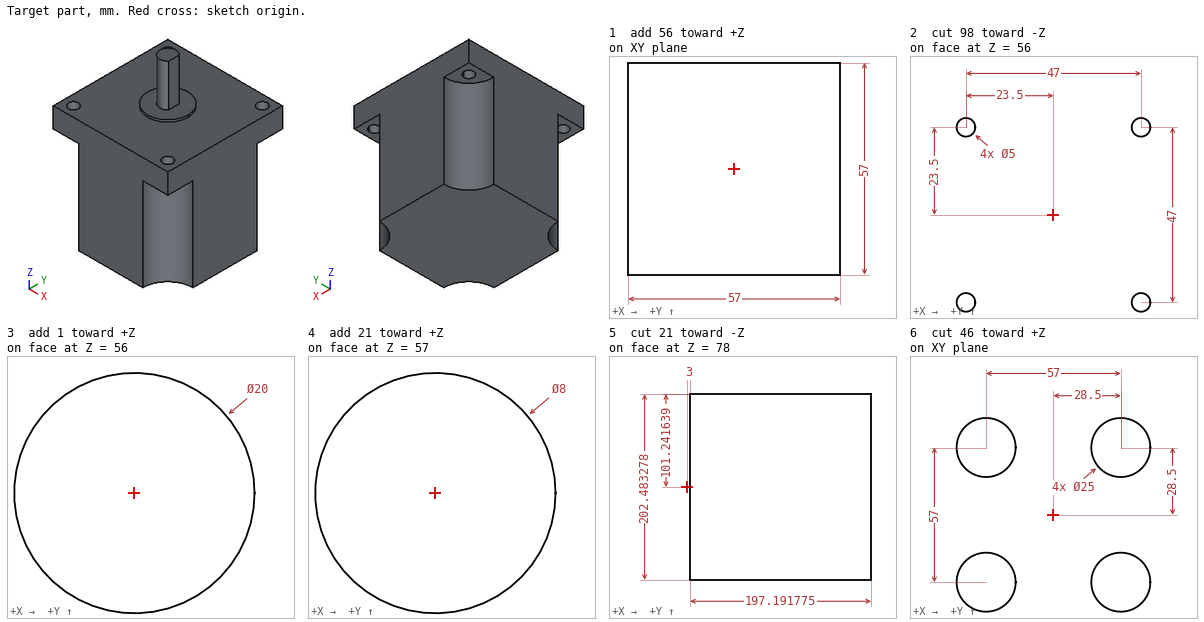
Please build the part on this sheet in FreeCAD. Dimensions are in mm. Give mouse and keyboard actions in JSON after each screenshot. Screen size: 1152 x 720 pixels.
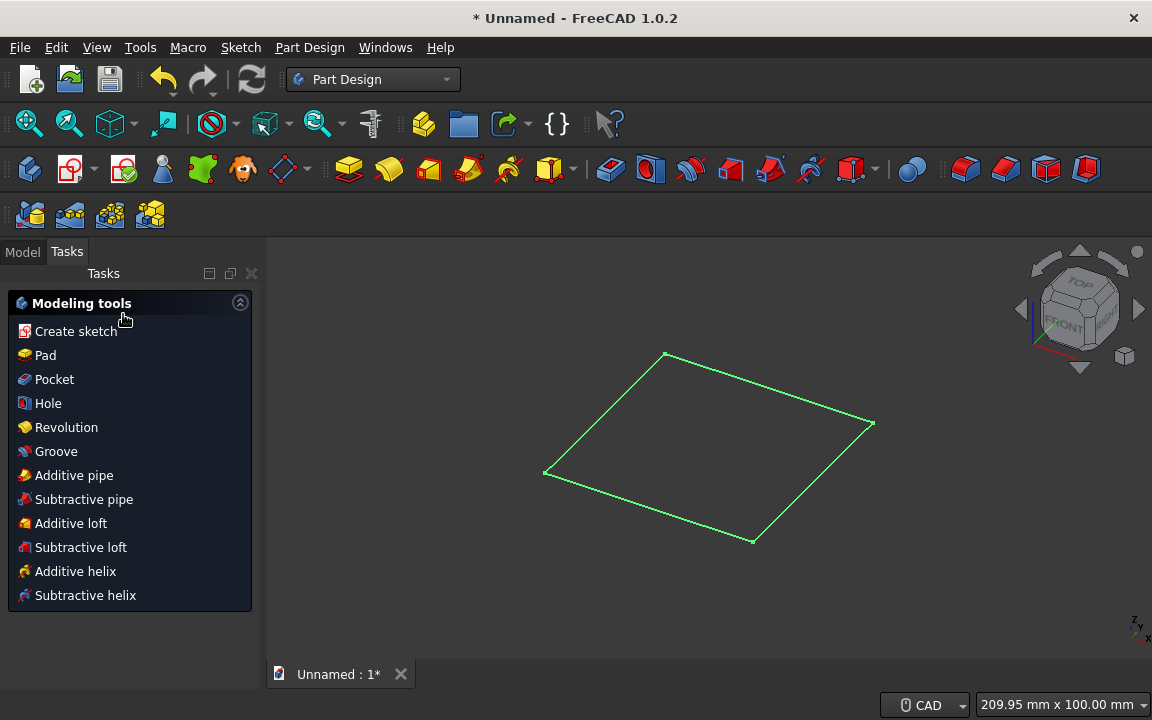
{"action": "left_click", "coordinate": [350, 170]}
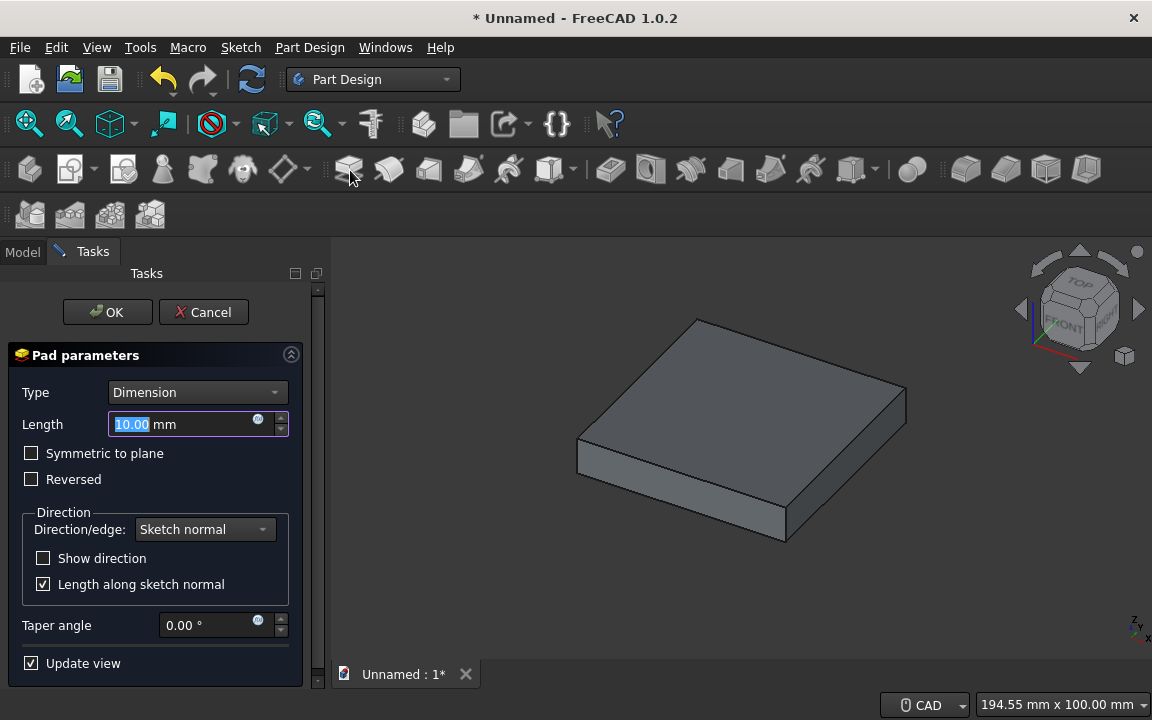
{"action": "type", "text": "56"}
{"action": "key", "text": "Tab"}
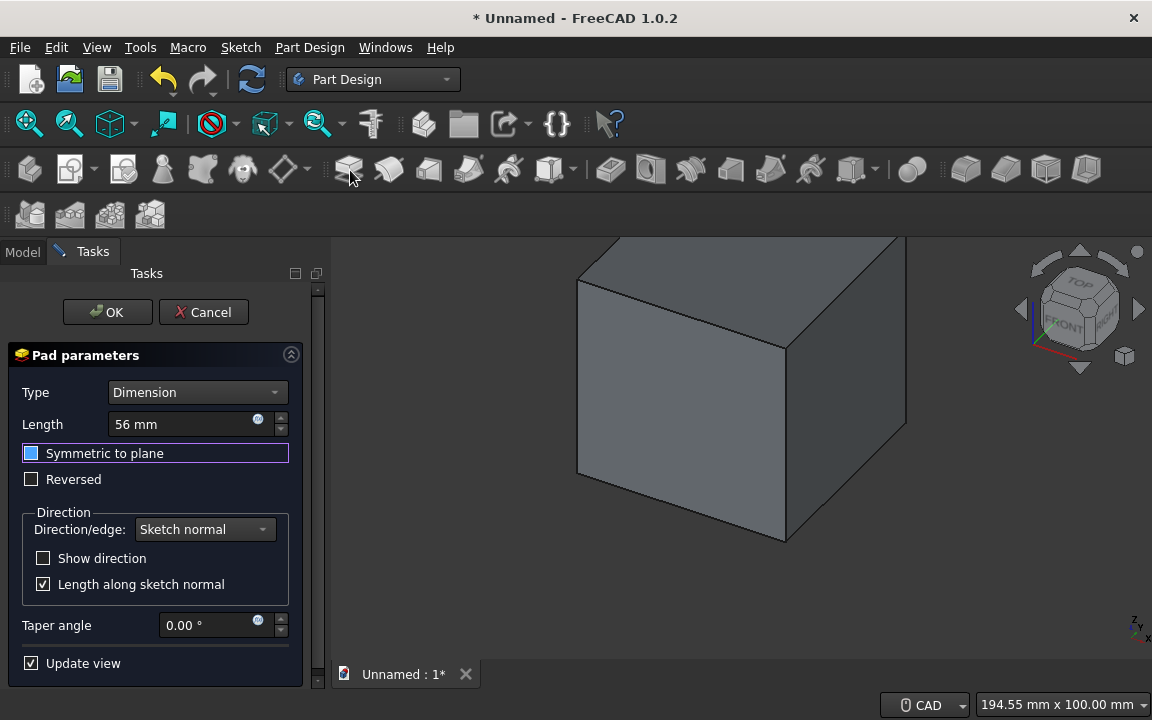
{"action": "left_click", "coordinate": [108, 312]}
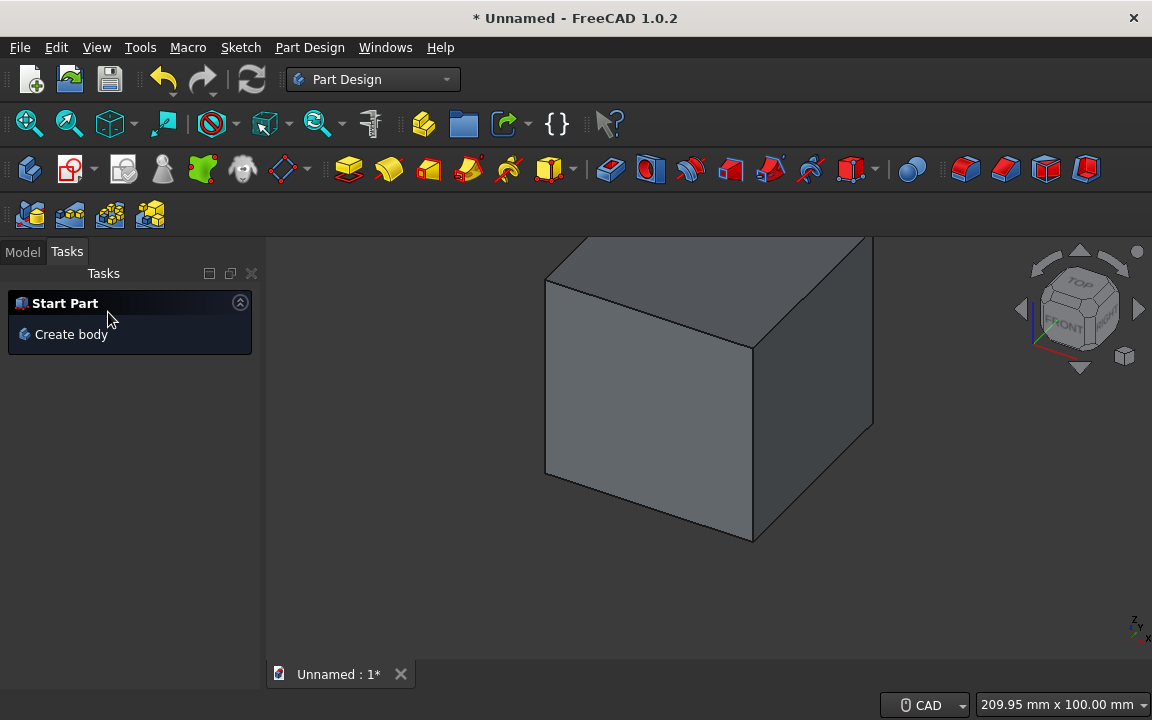
{"action": "left_click", "coordinate": [30, 124]}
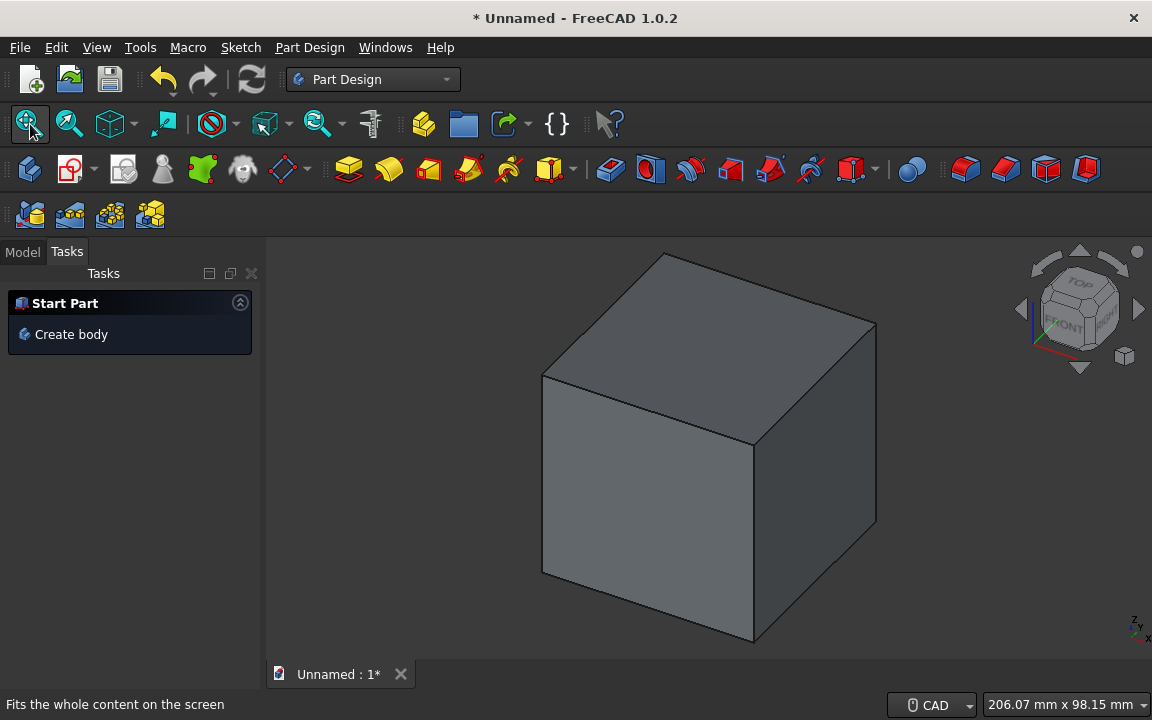
{"action": "left_click", "coordinate": [709, 348]}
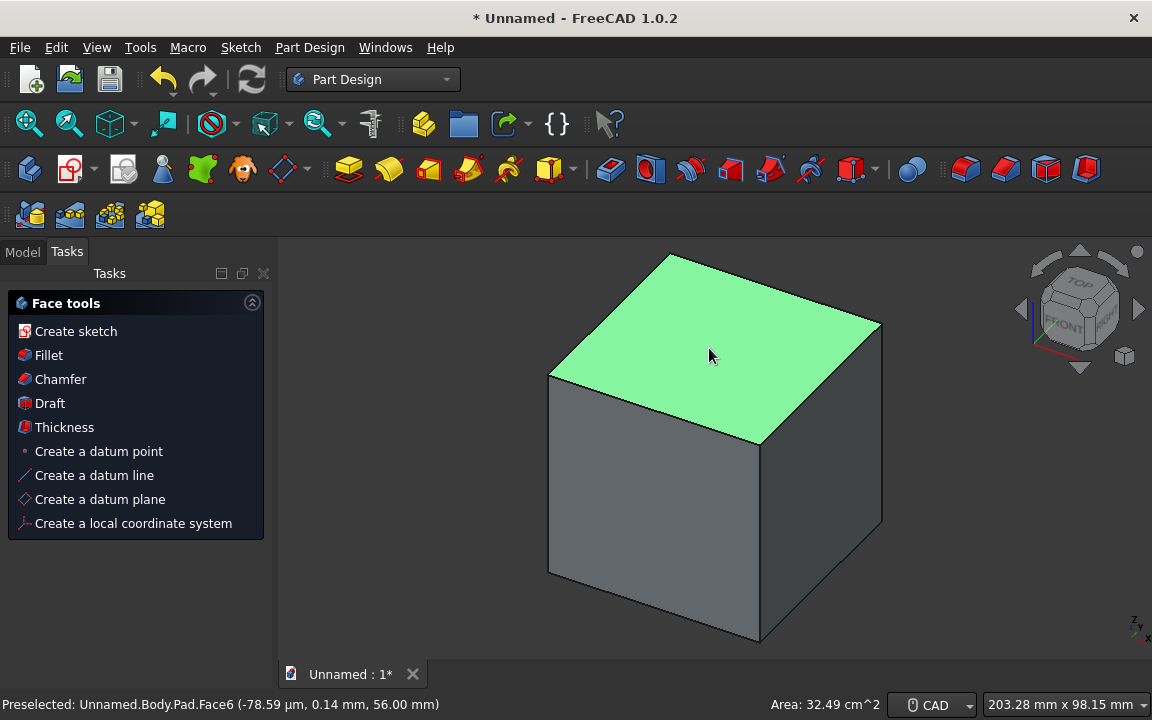
{"action": "left_click", "coordinate": [70, 170]}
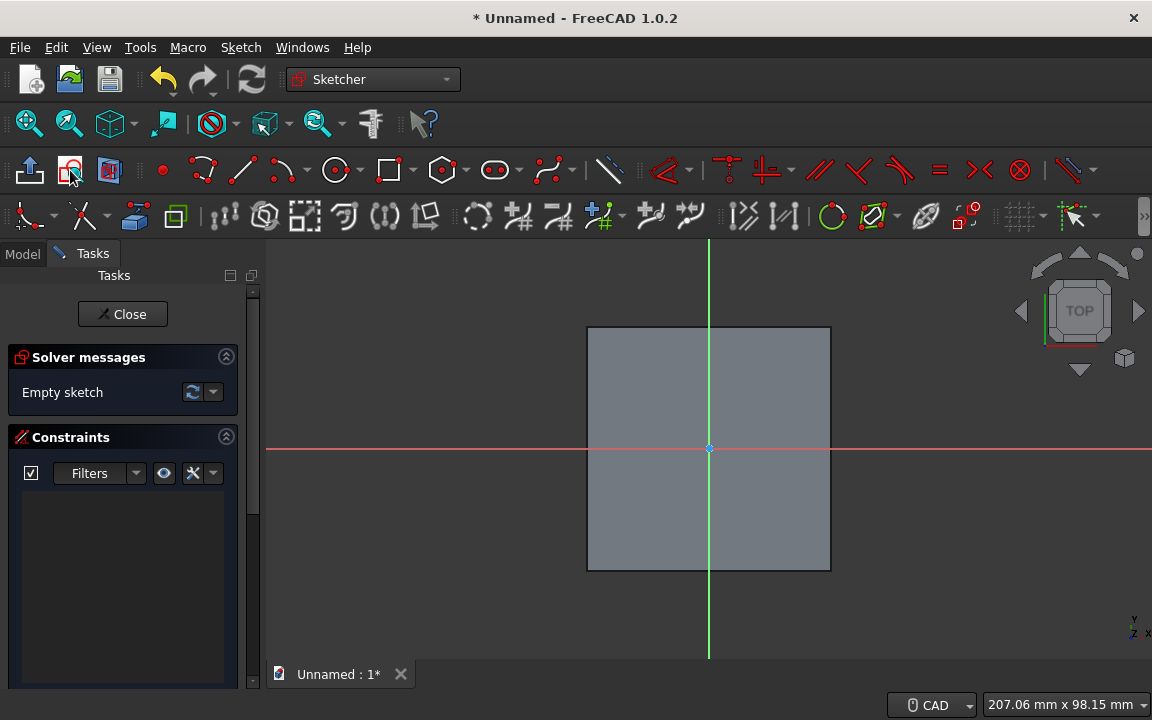
{"action": "left_click", "coordinate": [336, 170]}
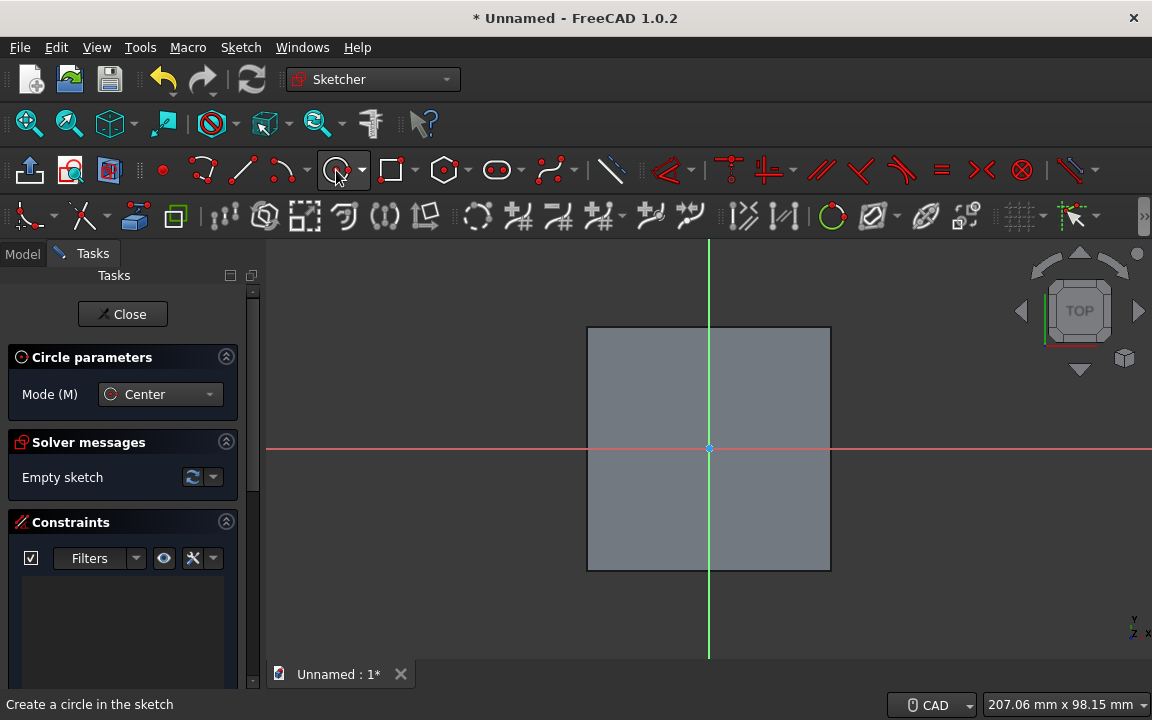
{"action": "scroll", "coordinate": [608, 348], "scroll_direction": "up", "scroll_amount": 4}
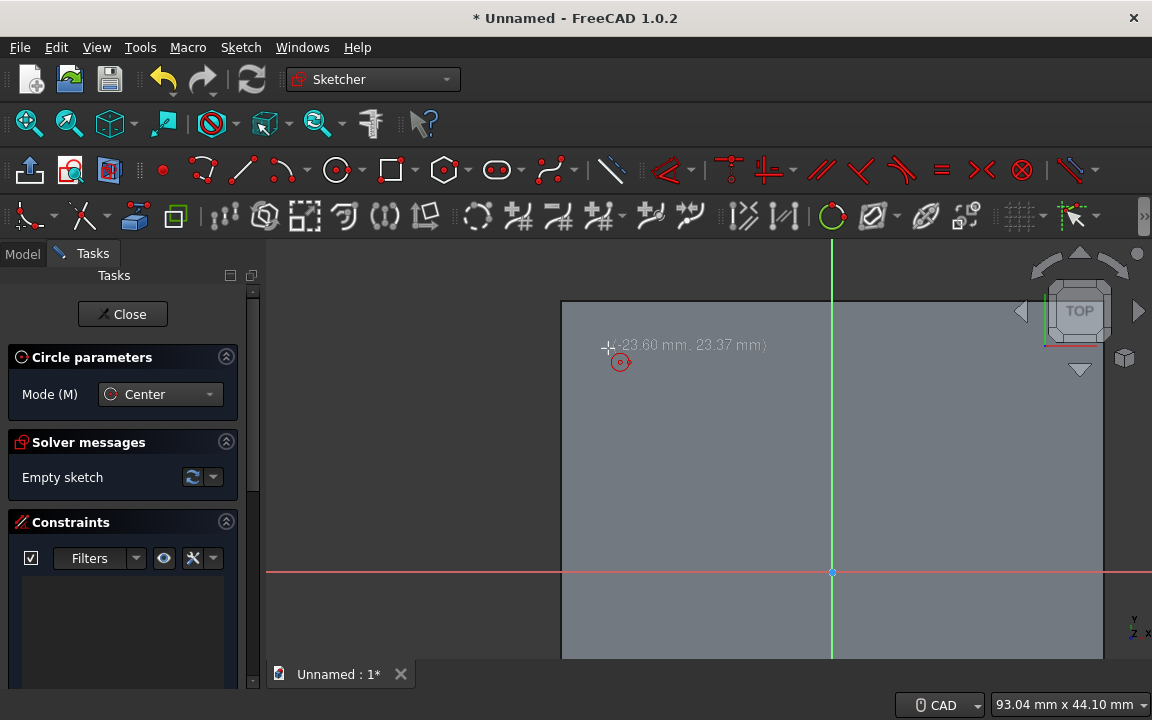
{"action": "left_click", "coordinate": [609, 349]}
{"action": "left_click", "coordinate": [625, 332]}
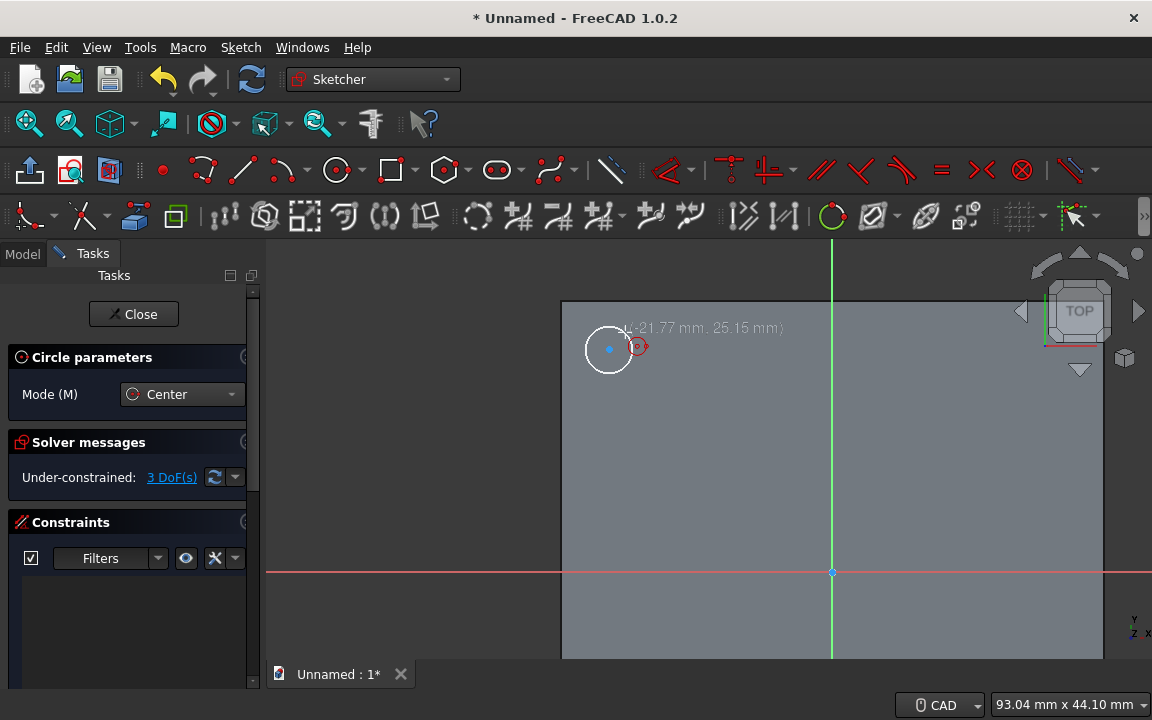
{"action": "scroll", "coordinate": [407, 299], "scroll_direction": "down", "scroll_amount": 3}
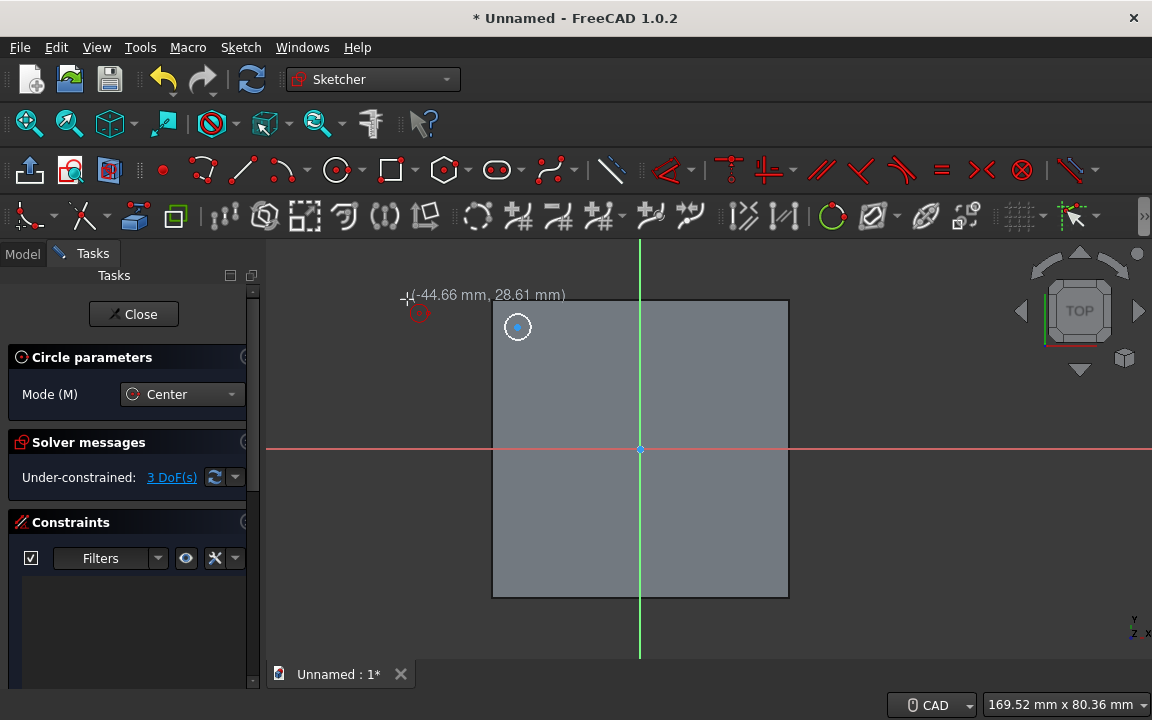
{"action": "scroll", "coordinate": [763, 326], "scroll_direction": "up", "scroll_amount": 3}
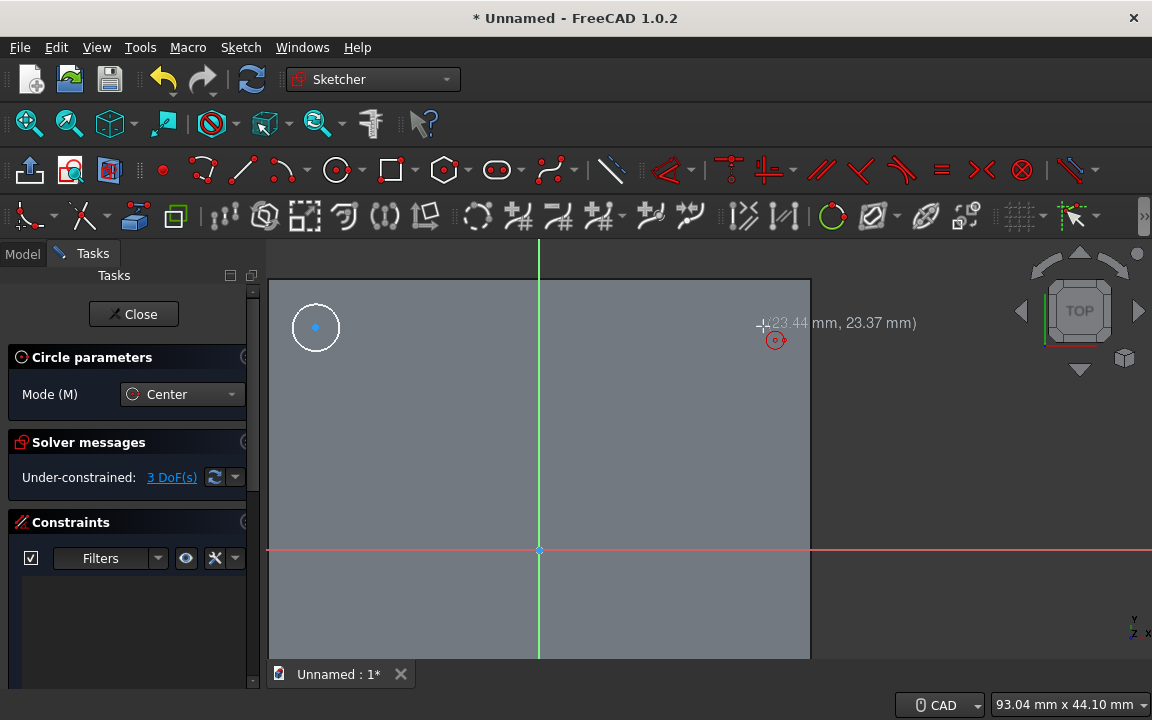
{"action": "left_click", "coordinate": [763, 326]}
{"action": "left_click", "coordinate": [780, 310]}